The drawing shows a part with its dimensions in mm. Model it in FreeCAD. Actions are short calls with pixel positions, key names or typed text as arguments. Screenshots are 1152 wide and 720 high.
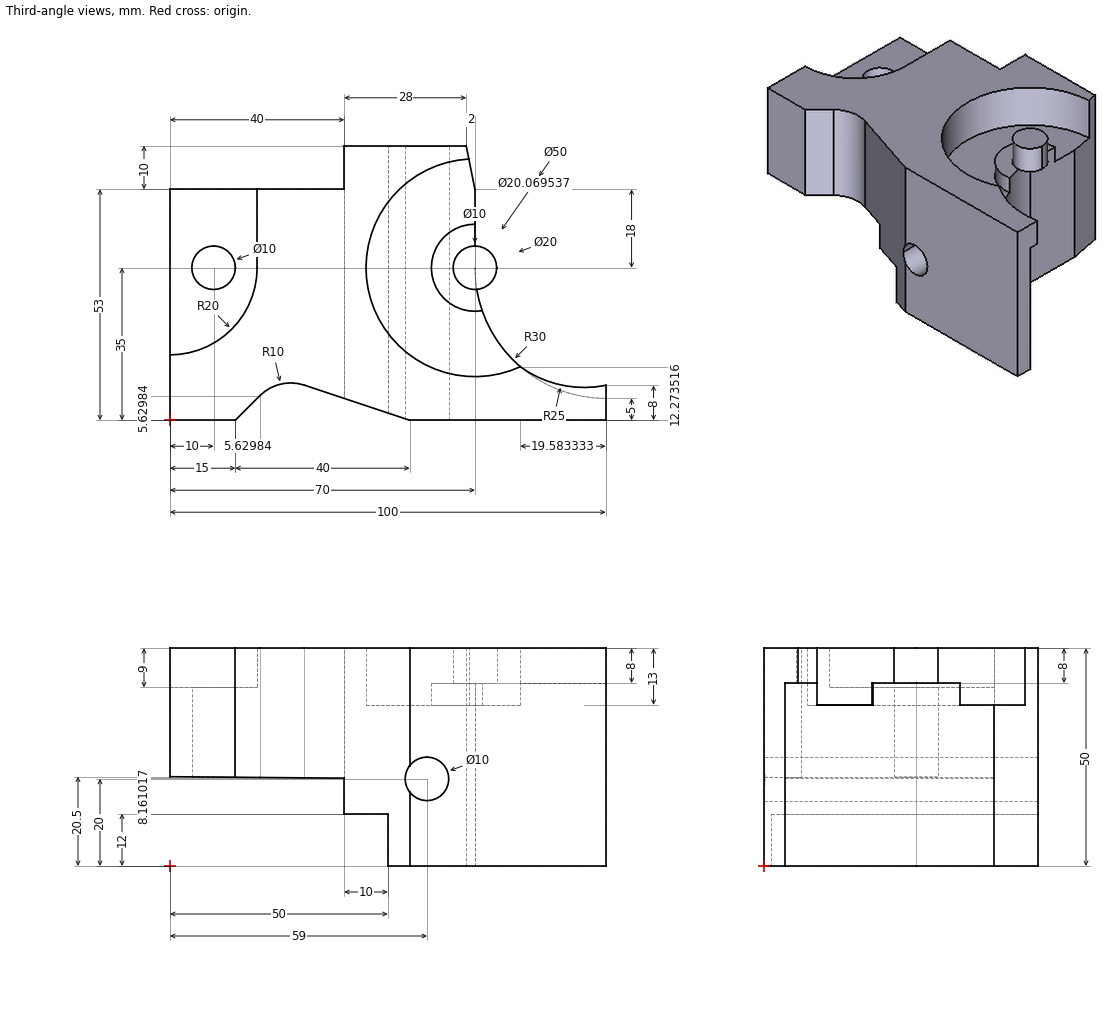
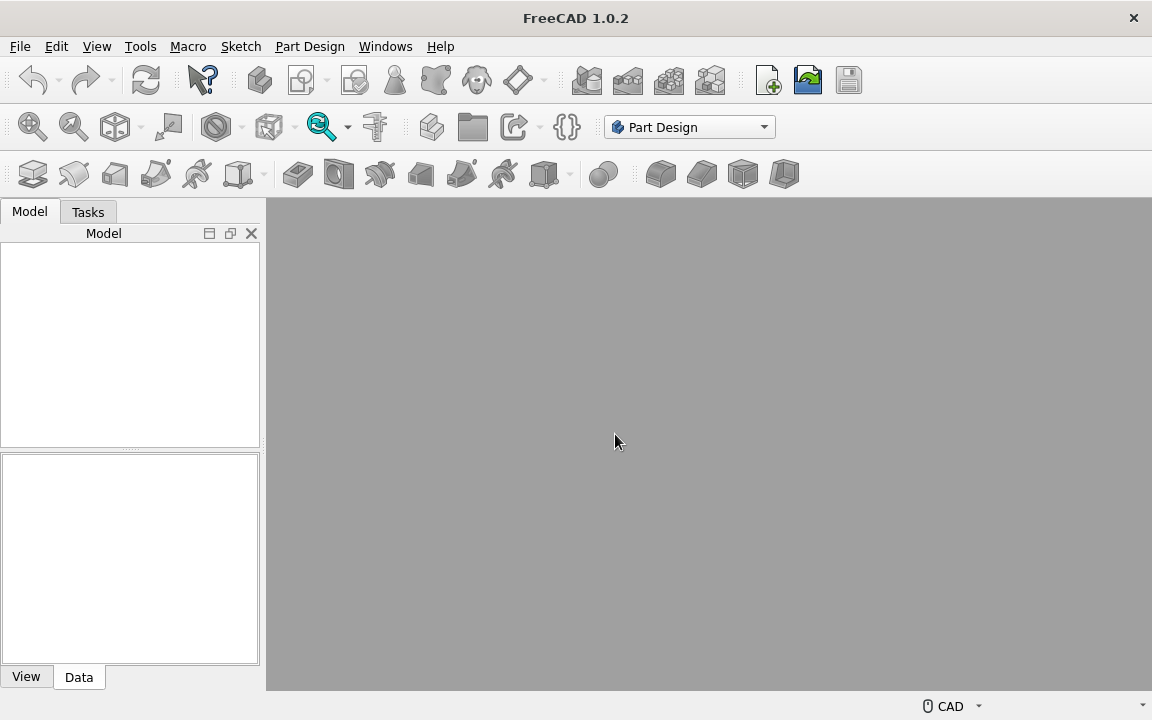
key(ctrl+n)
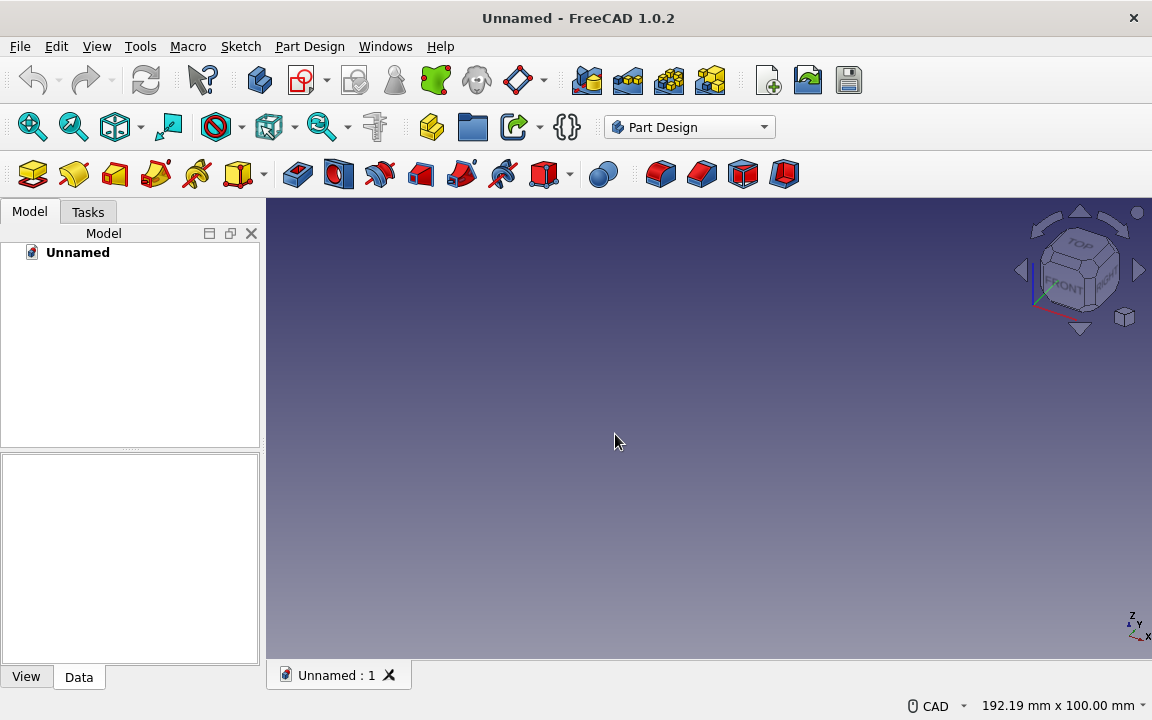
click(300, 80)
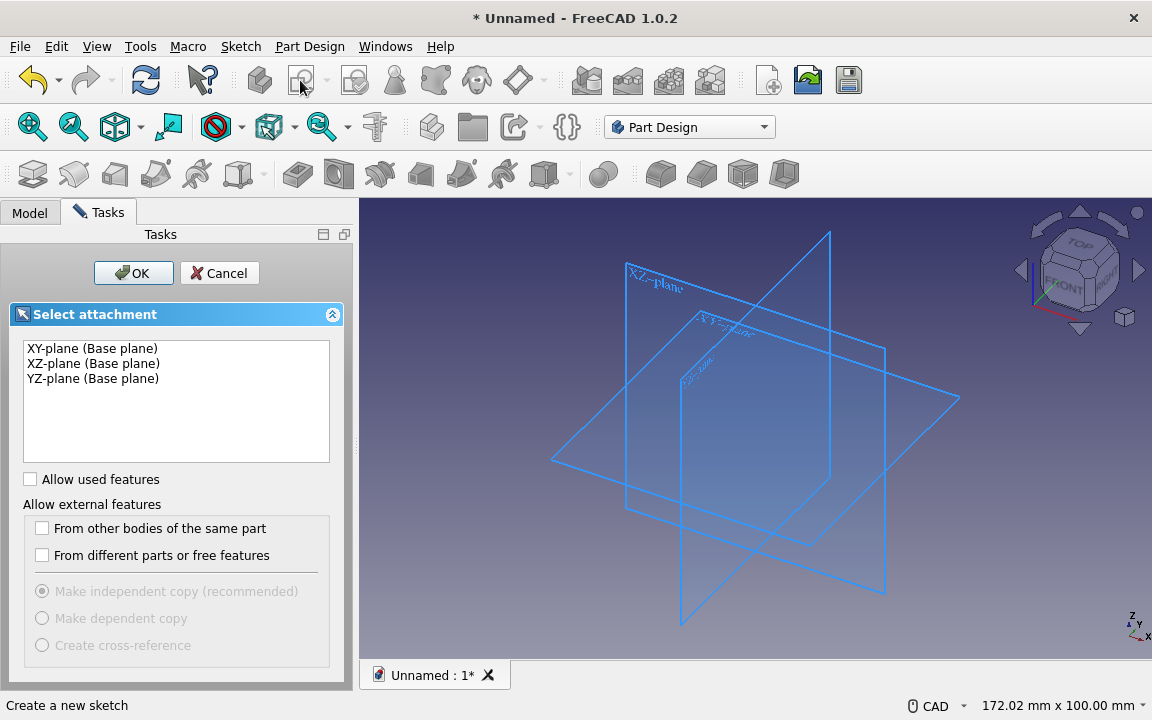
click(84, 348)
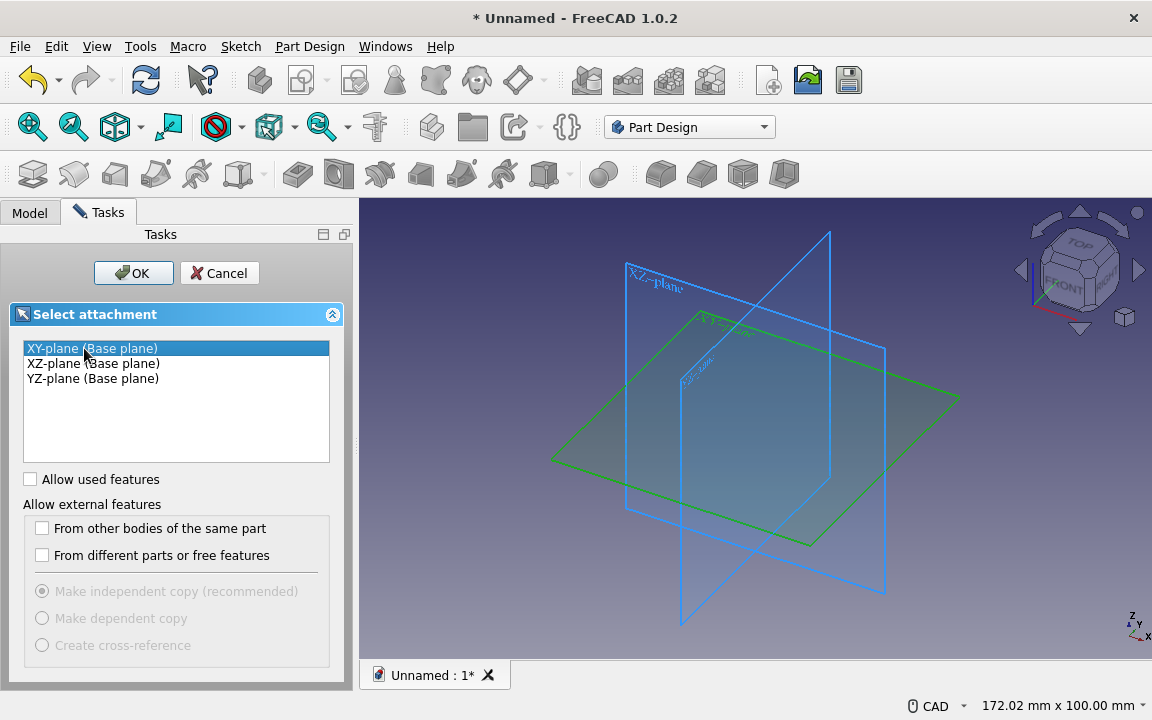
click(134, 273)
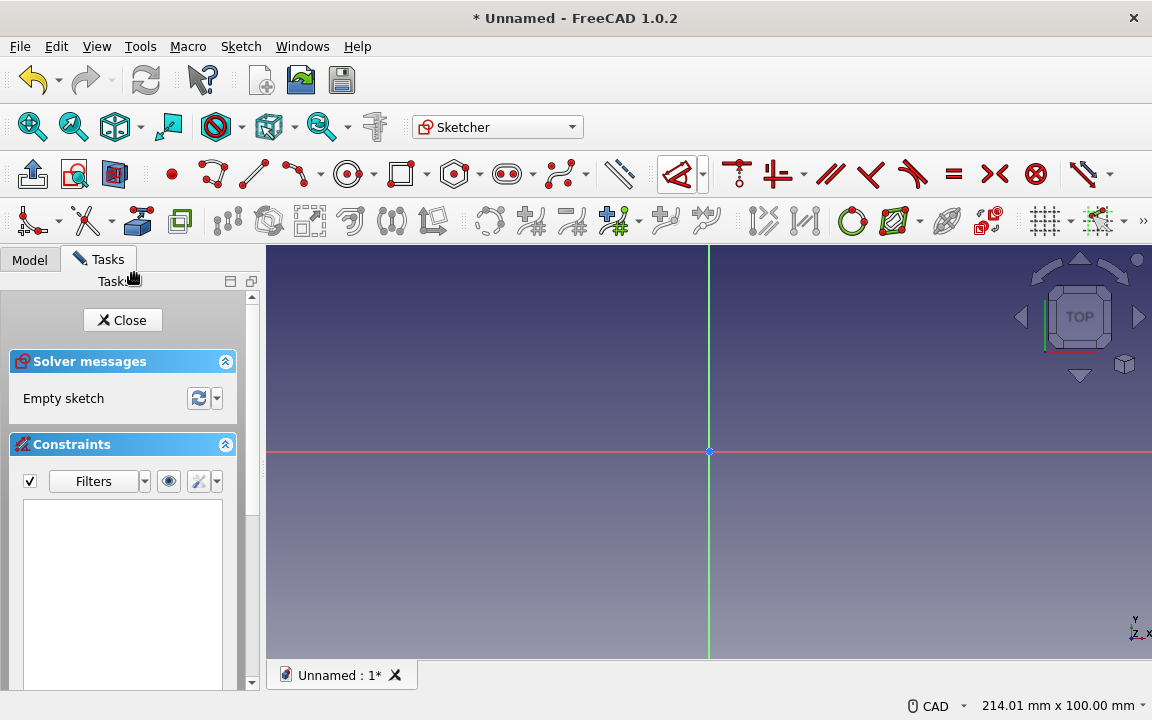
scroll(294, 631, down, 2)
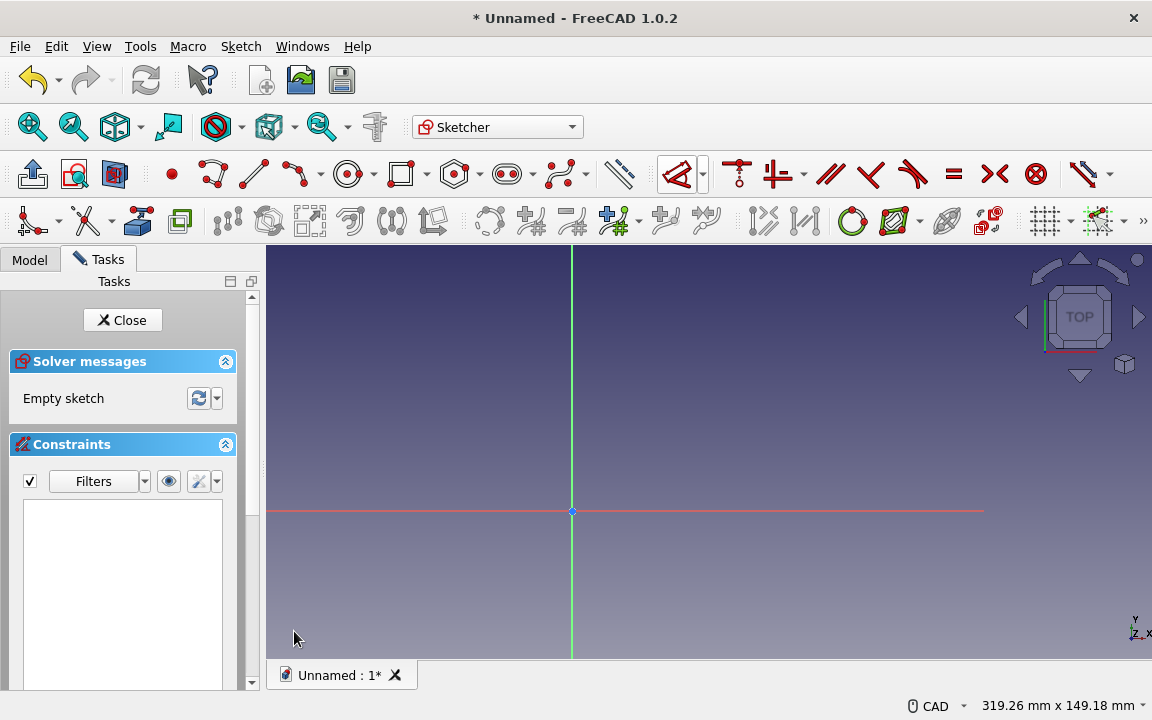
scroll(854, 367, up, 2)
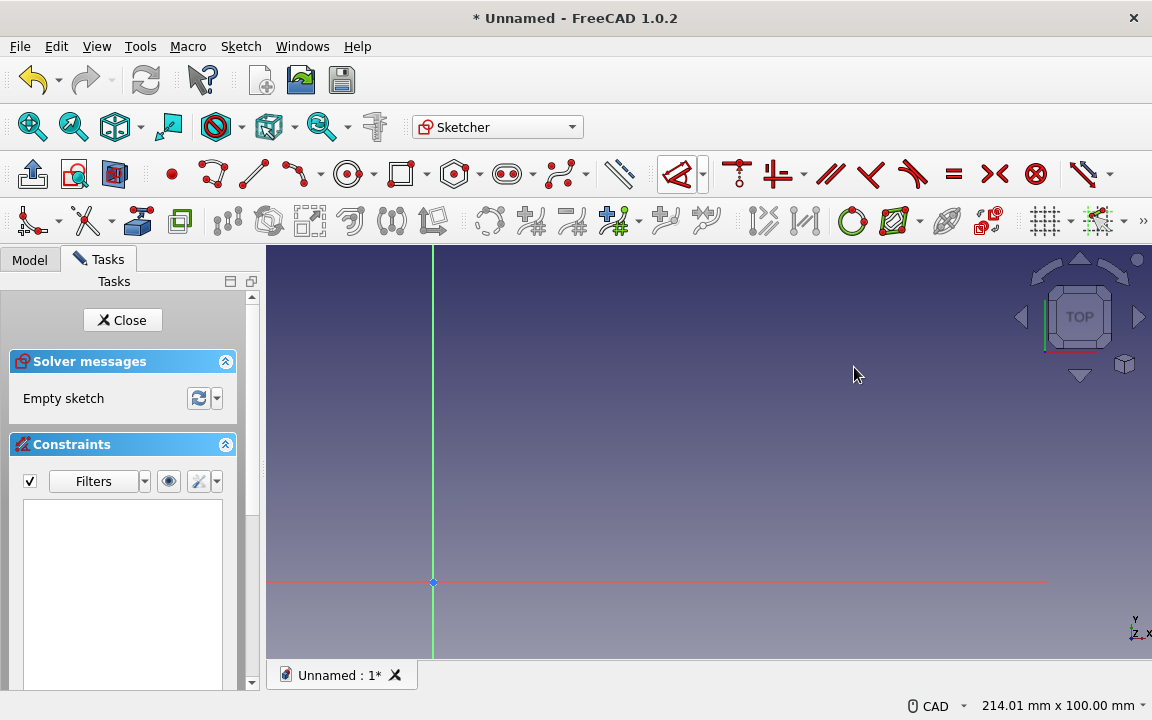
click(213, 174)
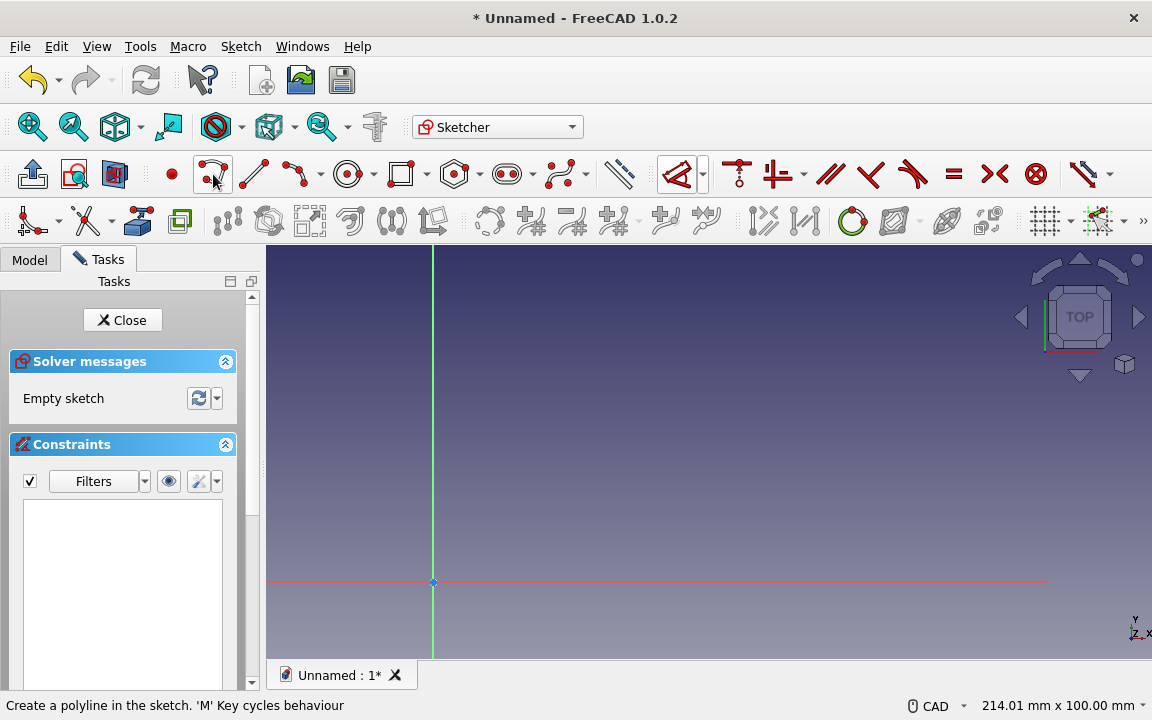
click(723, 437)
click(723, 363)
click(715, 321)
click(599, 321)
click(599, 363)
click(433, 363)
click(433, 582)
click(847, 573)
click(847, 561)
right_click(847, 561)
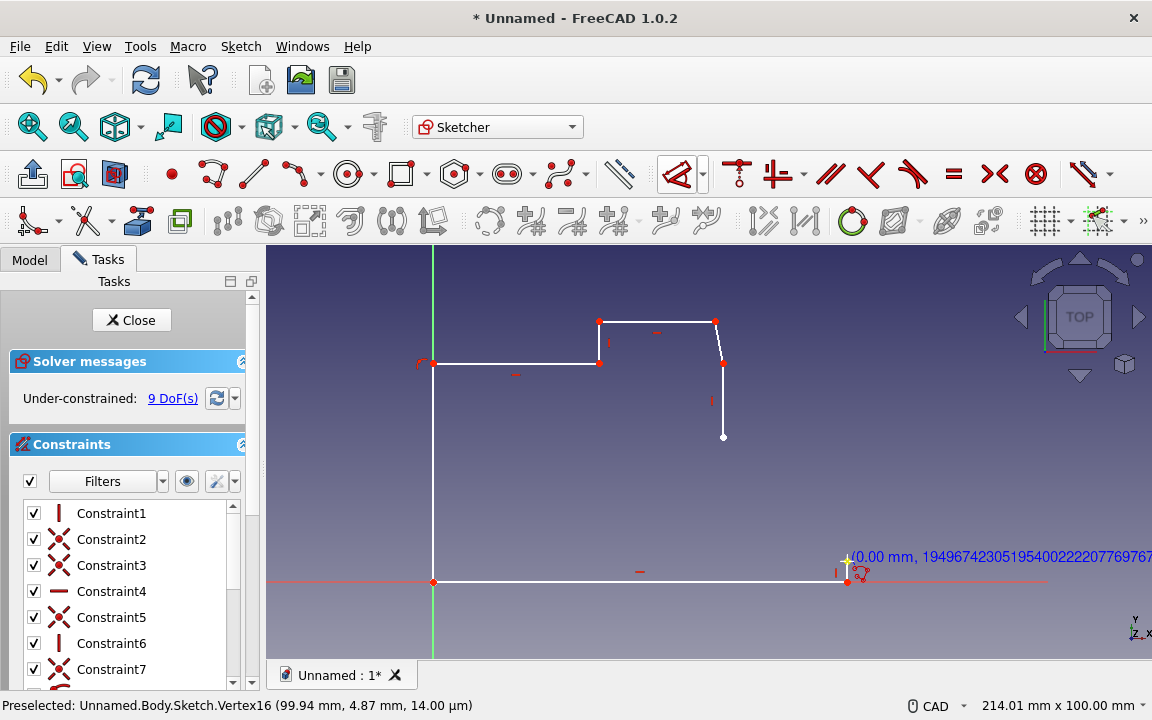
key(g)
key(3)
key(a)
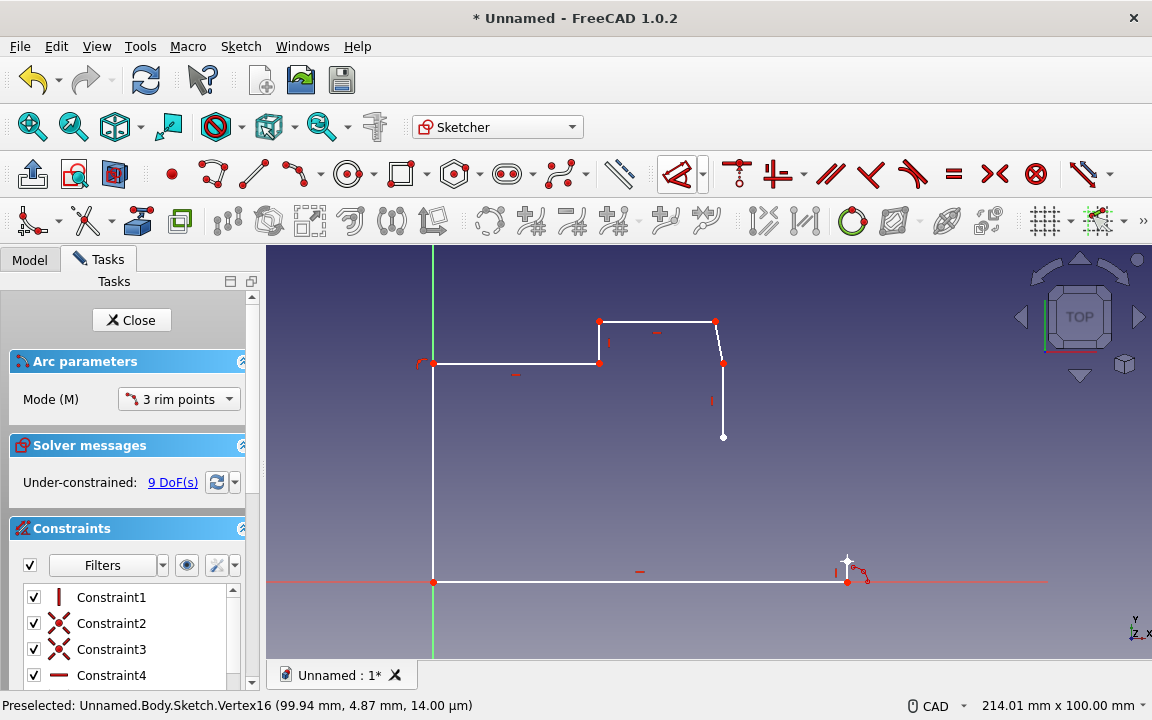
scroll(847, 561, up, 3)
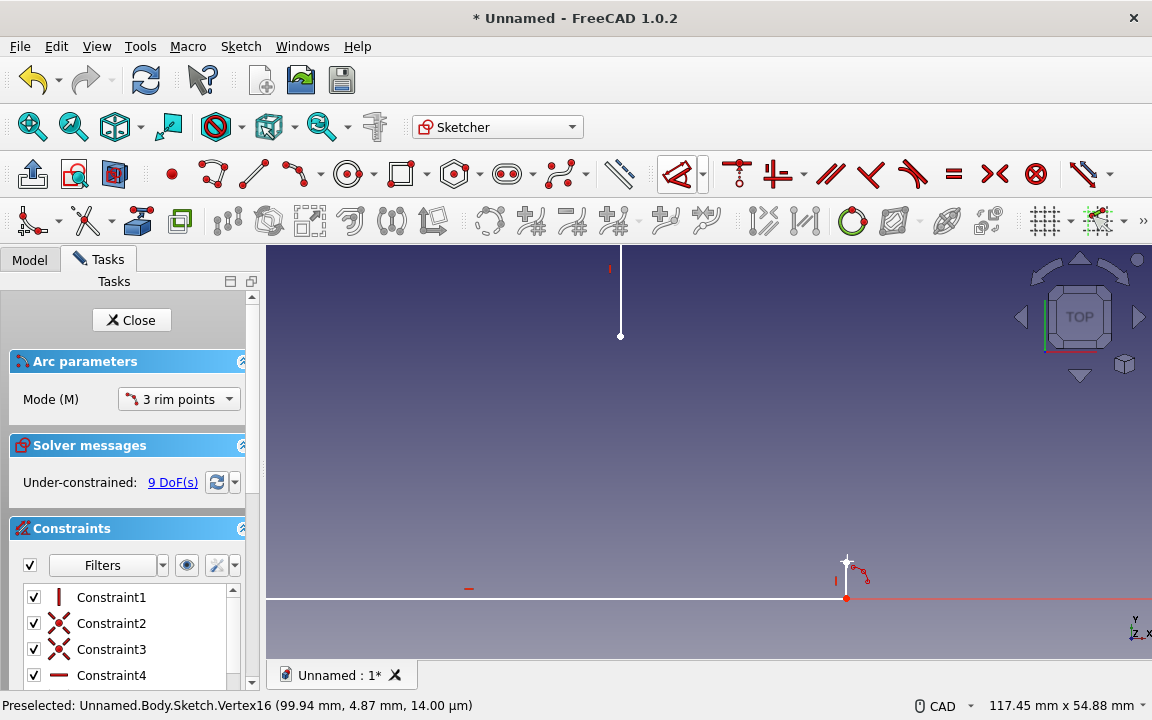
click(846, 562)
click(621, 336)
click(687, 495)
key(Escape)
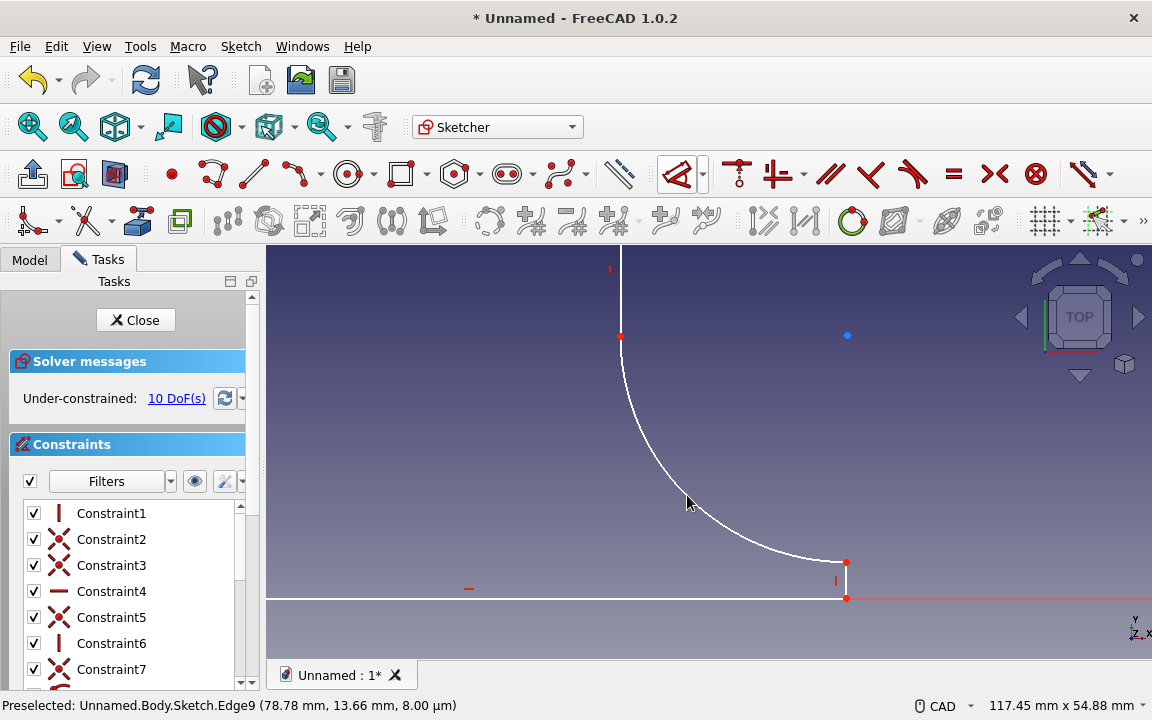
click(621, 296)